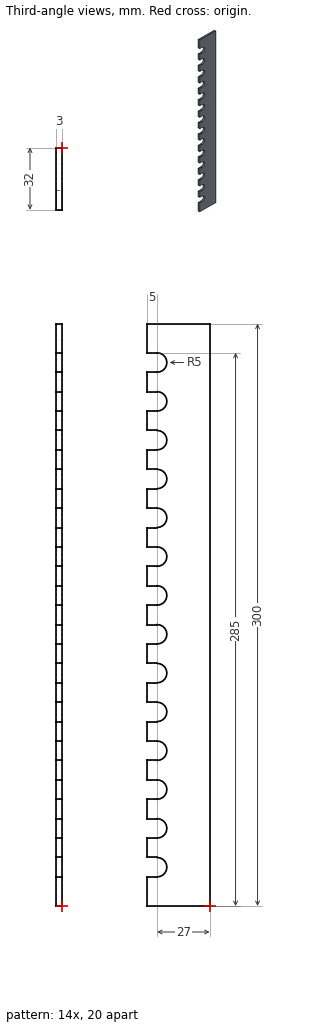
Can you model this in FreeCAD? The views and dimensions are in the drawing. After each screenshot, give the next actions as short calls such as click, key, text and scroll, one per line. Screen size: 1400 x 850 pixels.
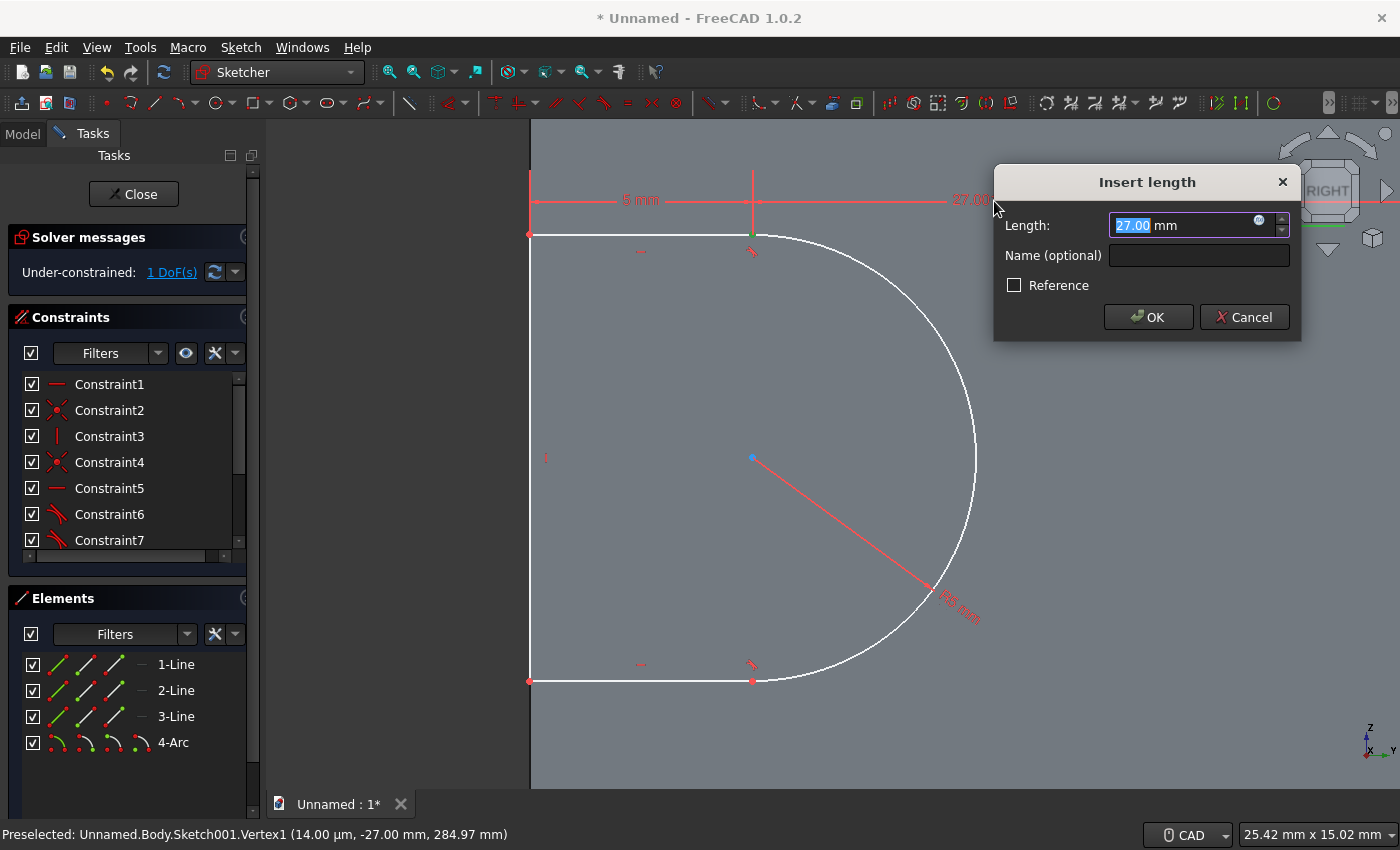
text(27)
key(Return)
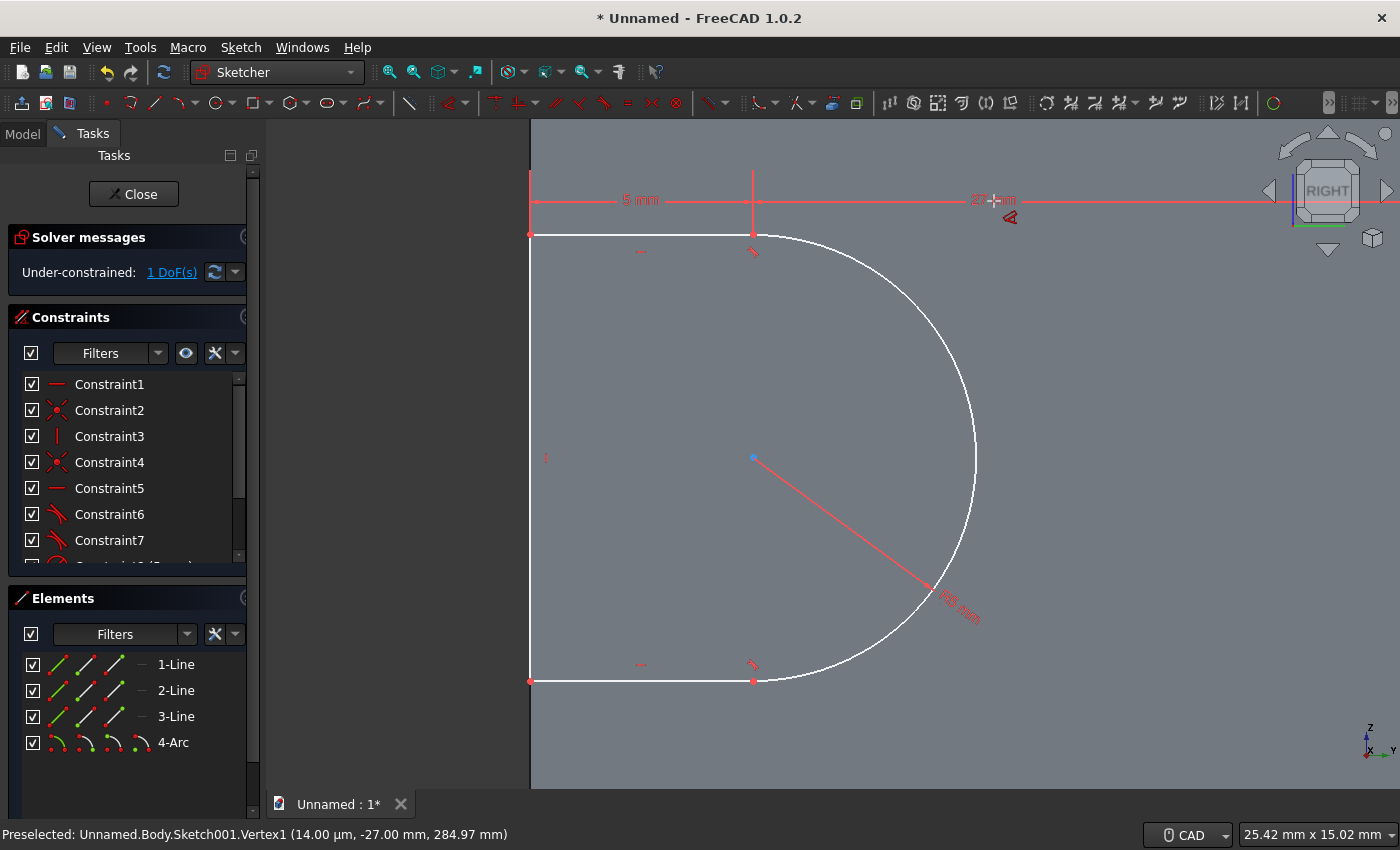
click(753, 235)
click(719, 498)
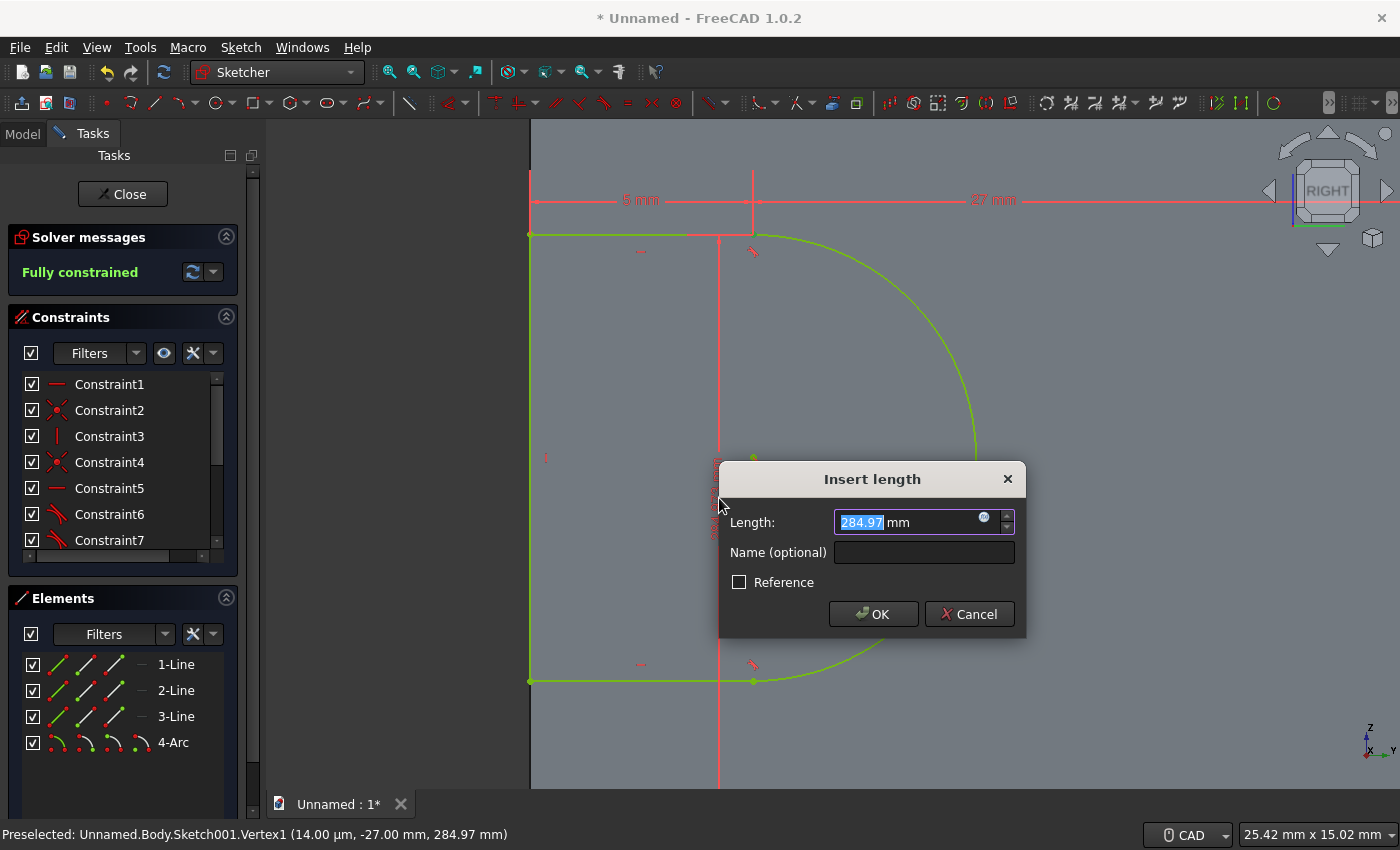
text(285)
key(Return)
key(Escape)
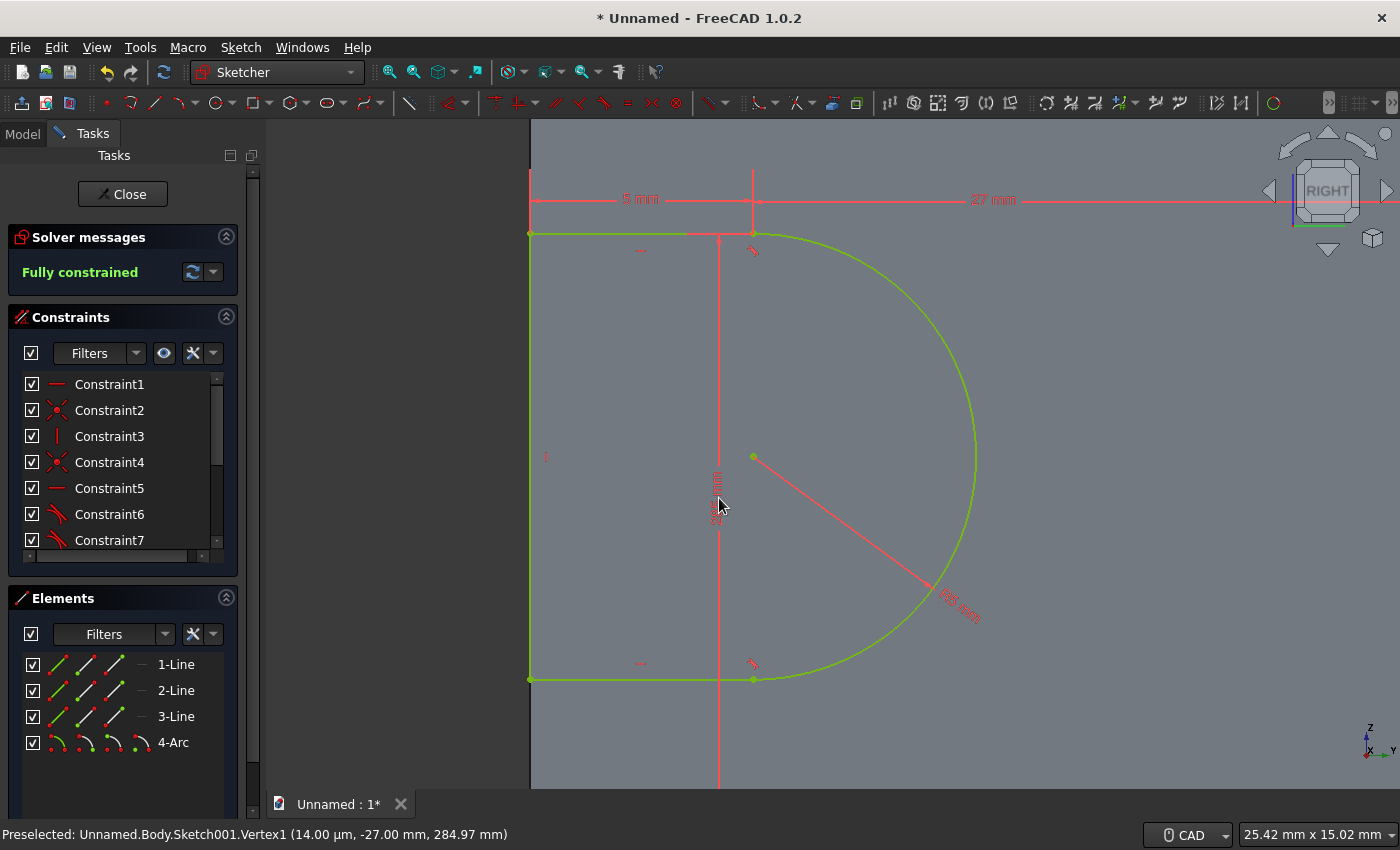
click(123, 194)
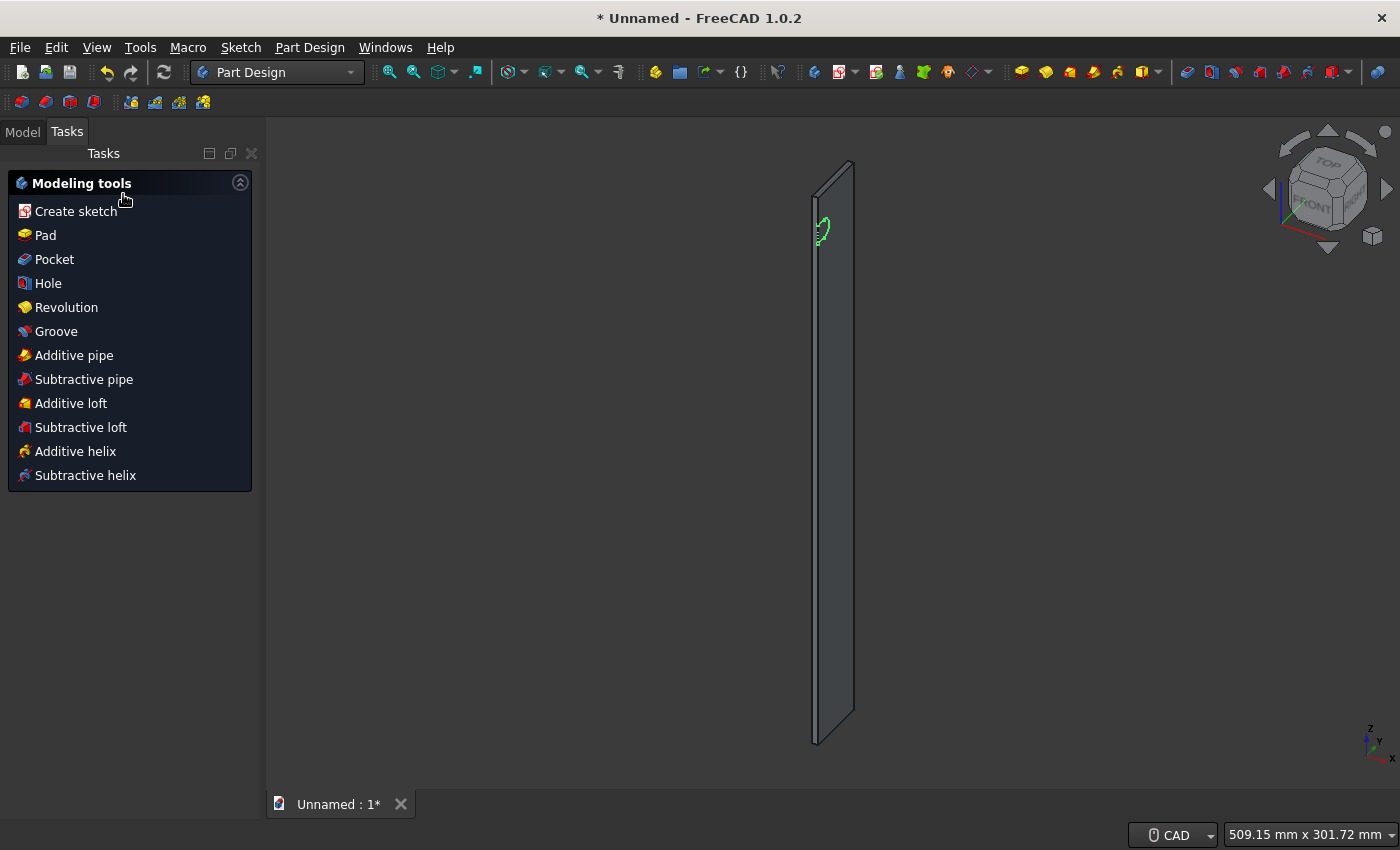
click(1188, 72)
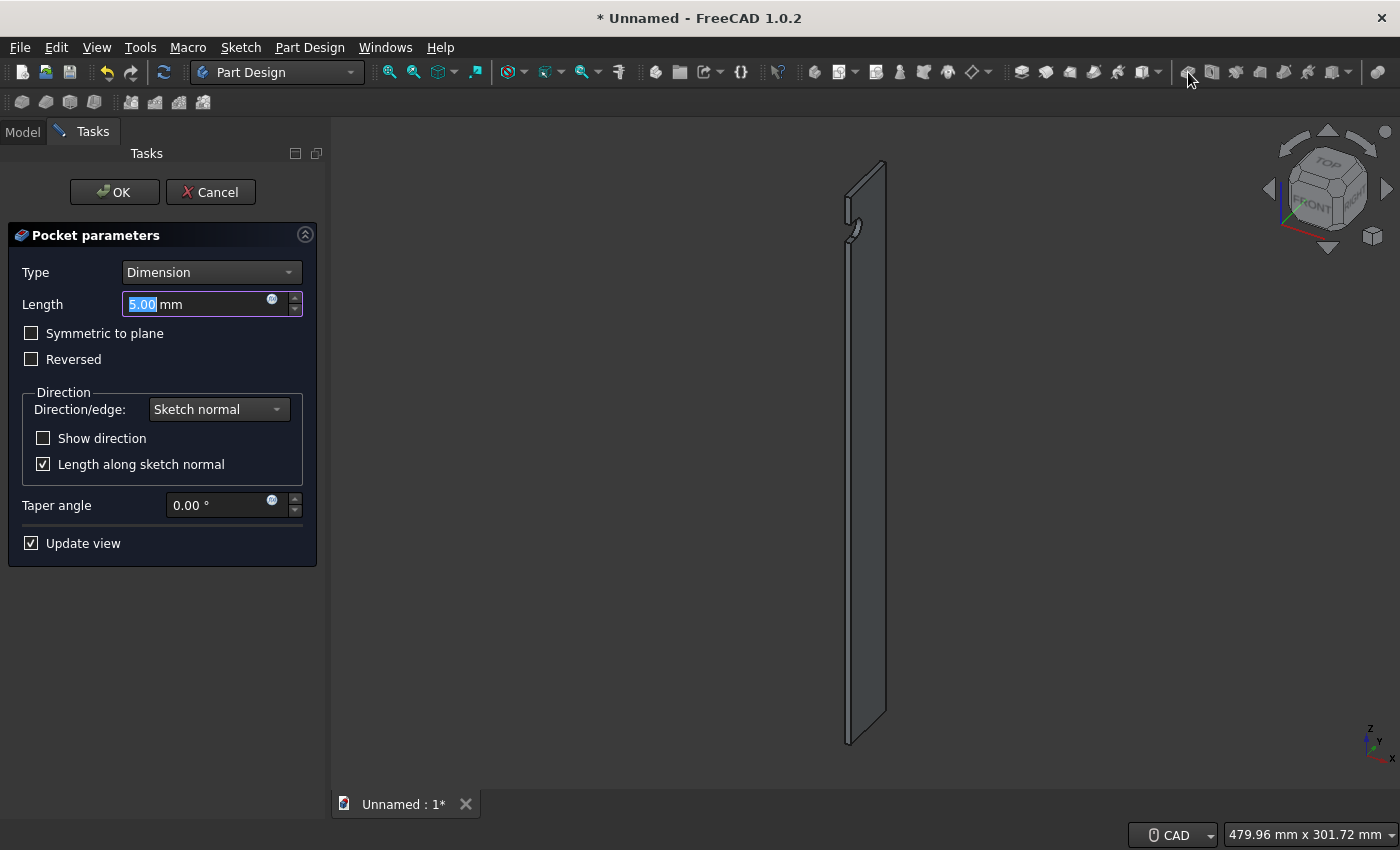
click(212, 272)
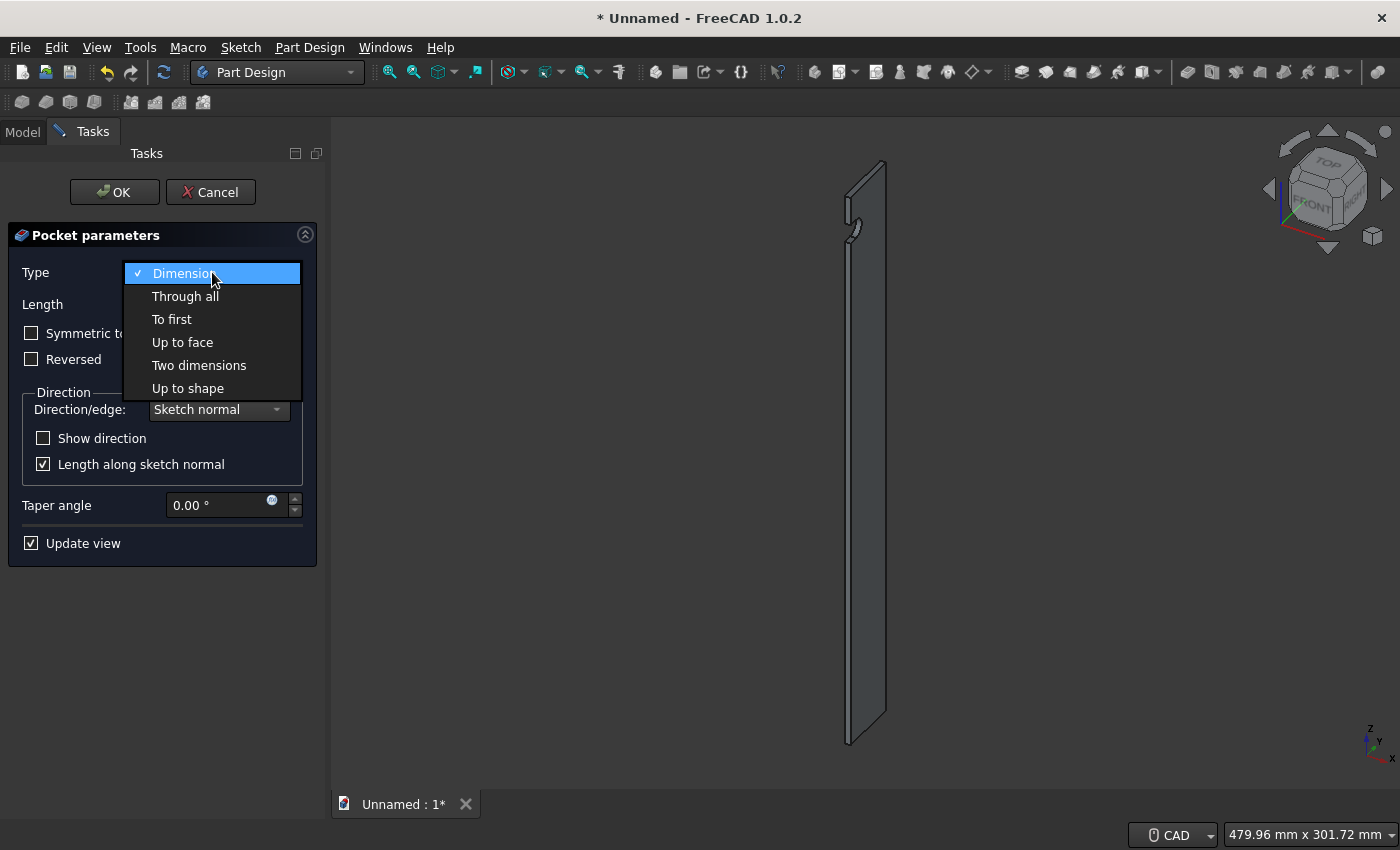
click(212, 296)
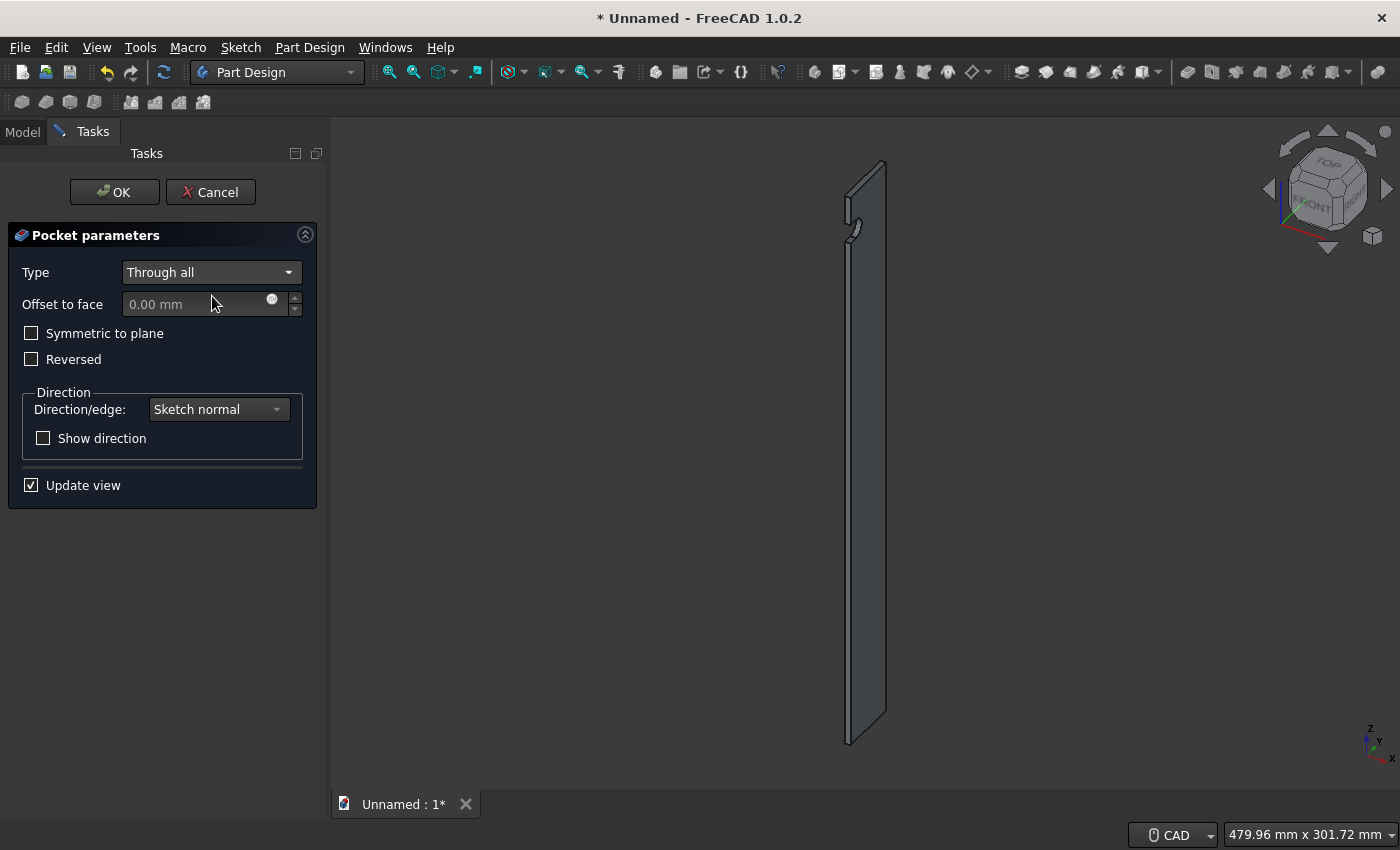
click(115, 192)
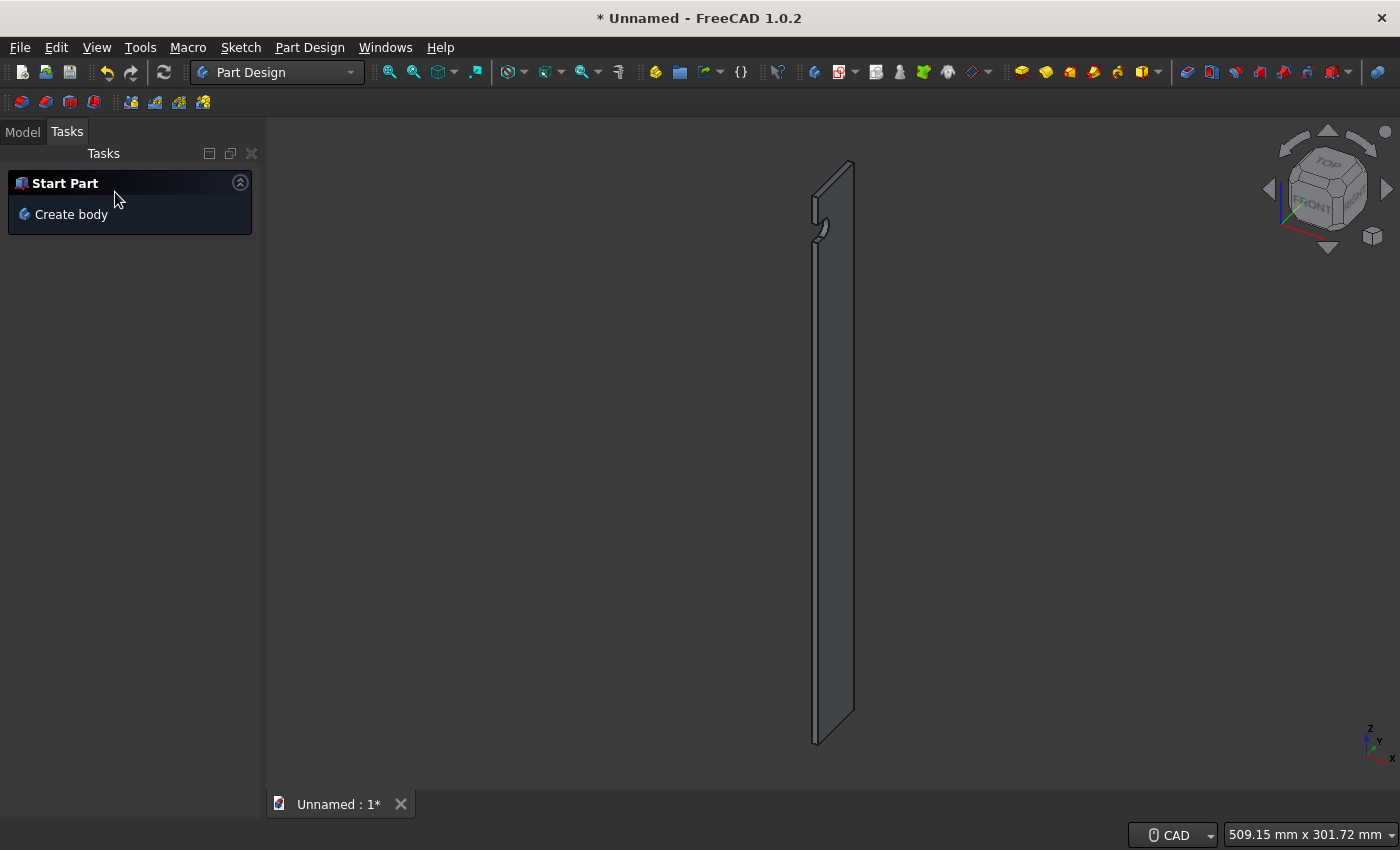
click(23, 131)